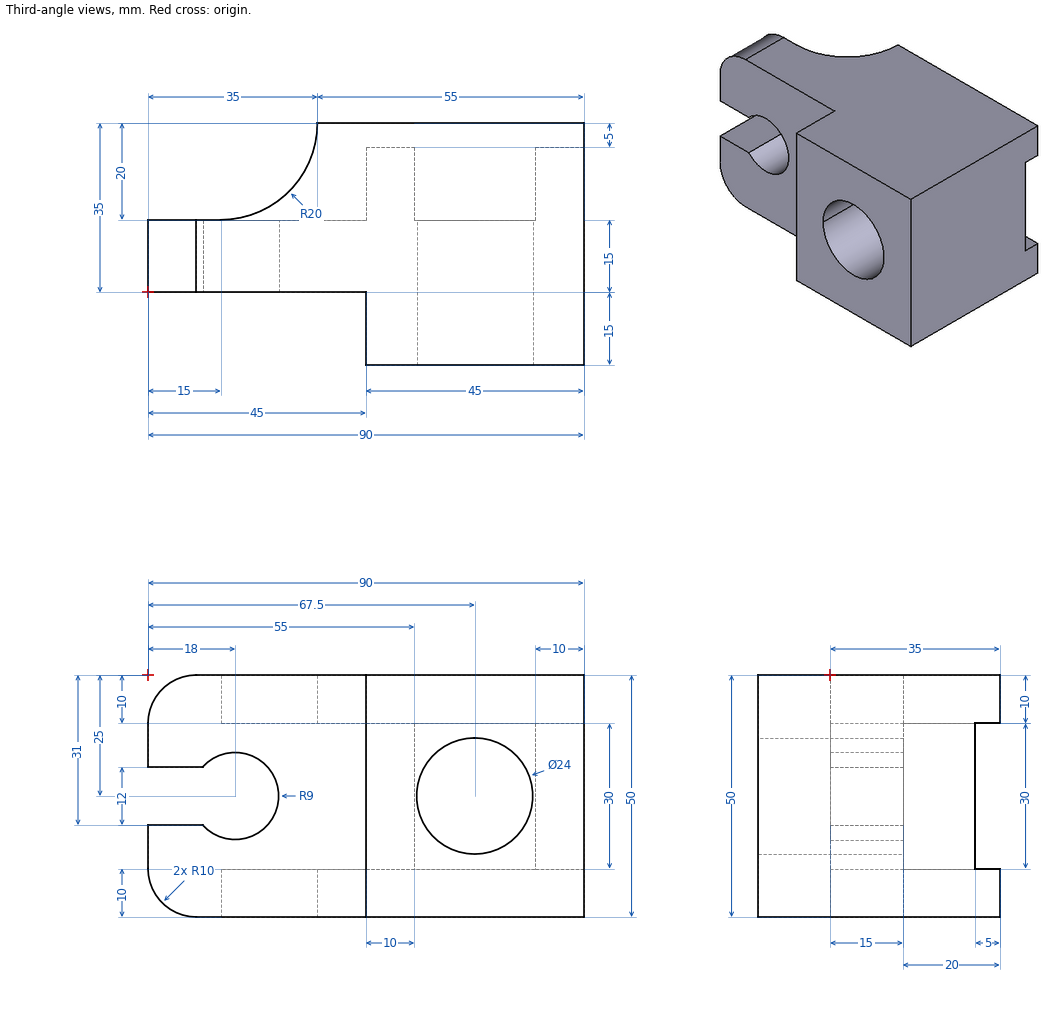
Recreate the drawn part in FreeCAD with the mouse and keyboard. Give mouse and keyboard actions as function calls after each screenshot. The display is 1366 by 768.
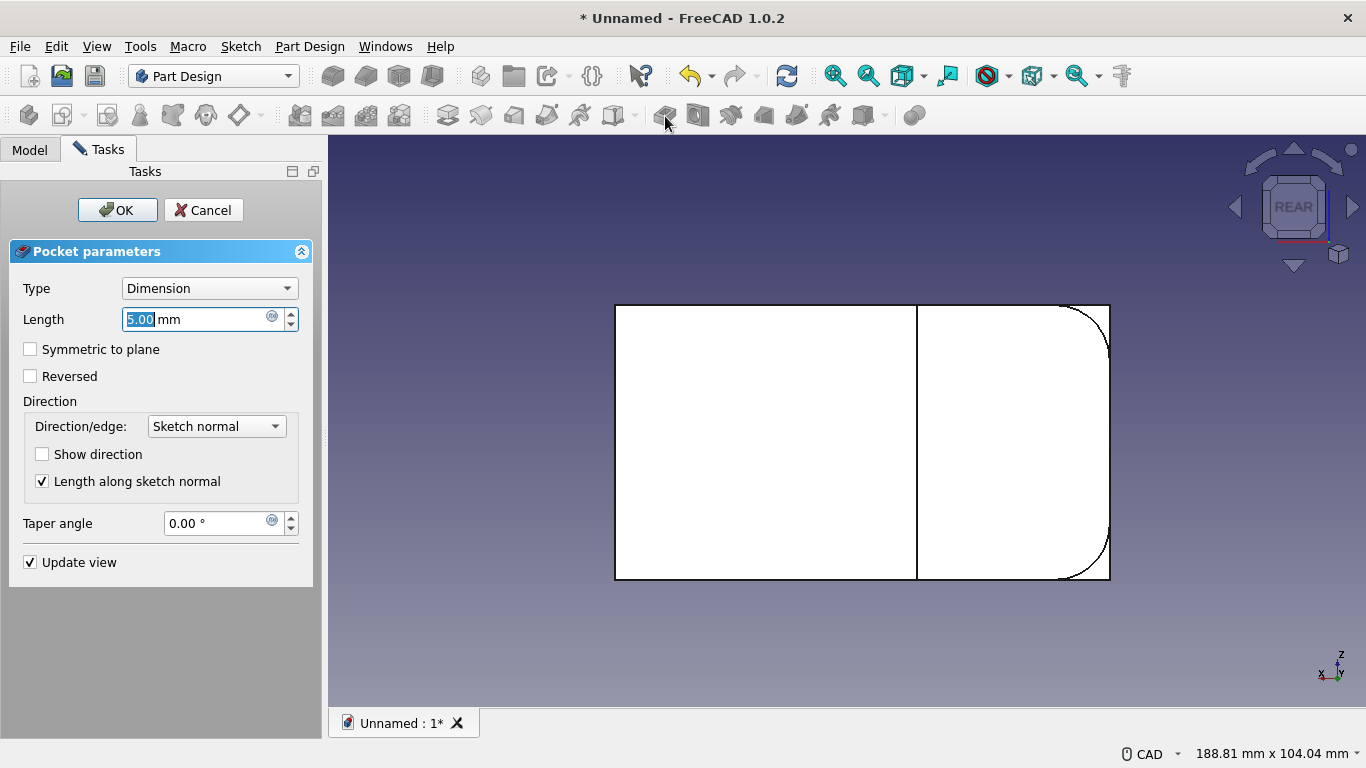
text(50)
key(Tab)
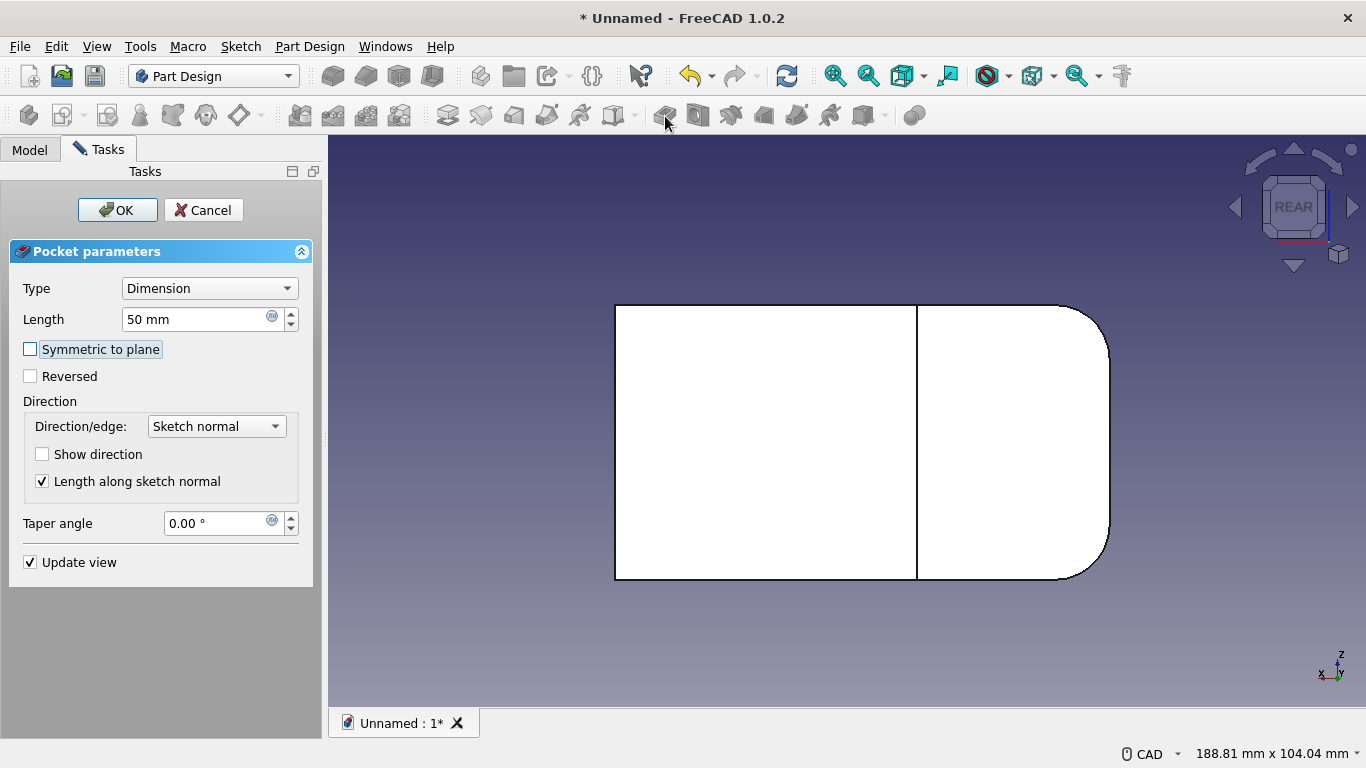
click(118, 210)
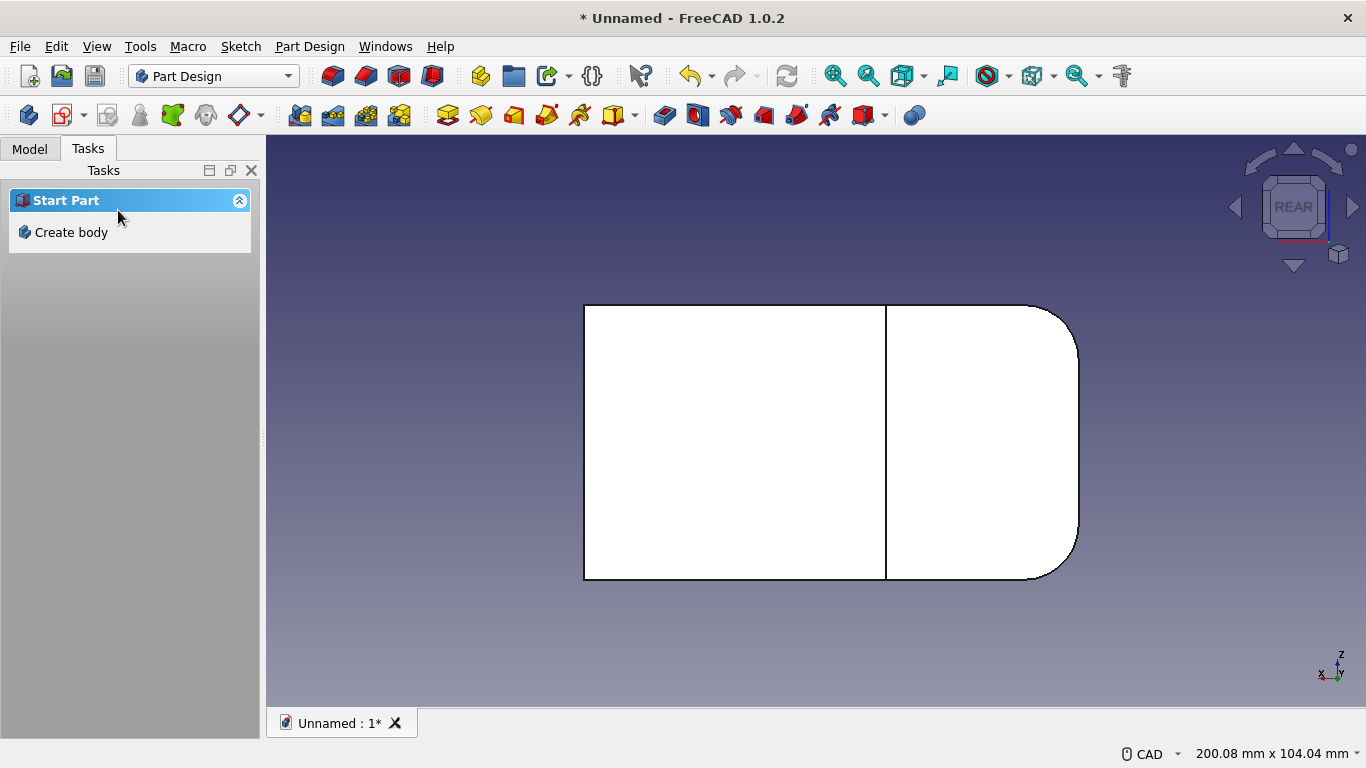
key(0)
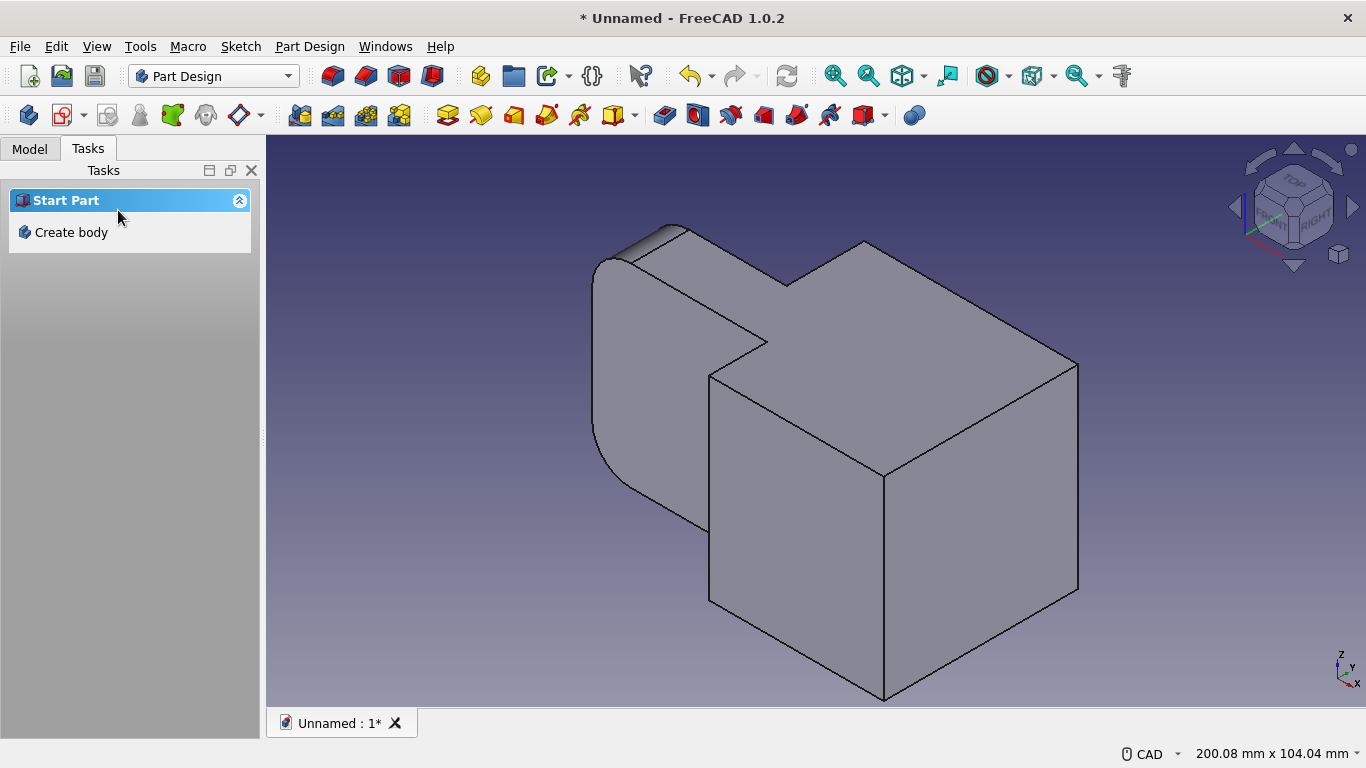
click(870, 355)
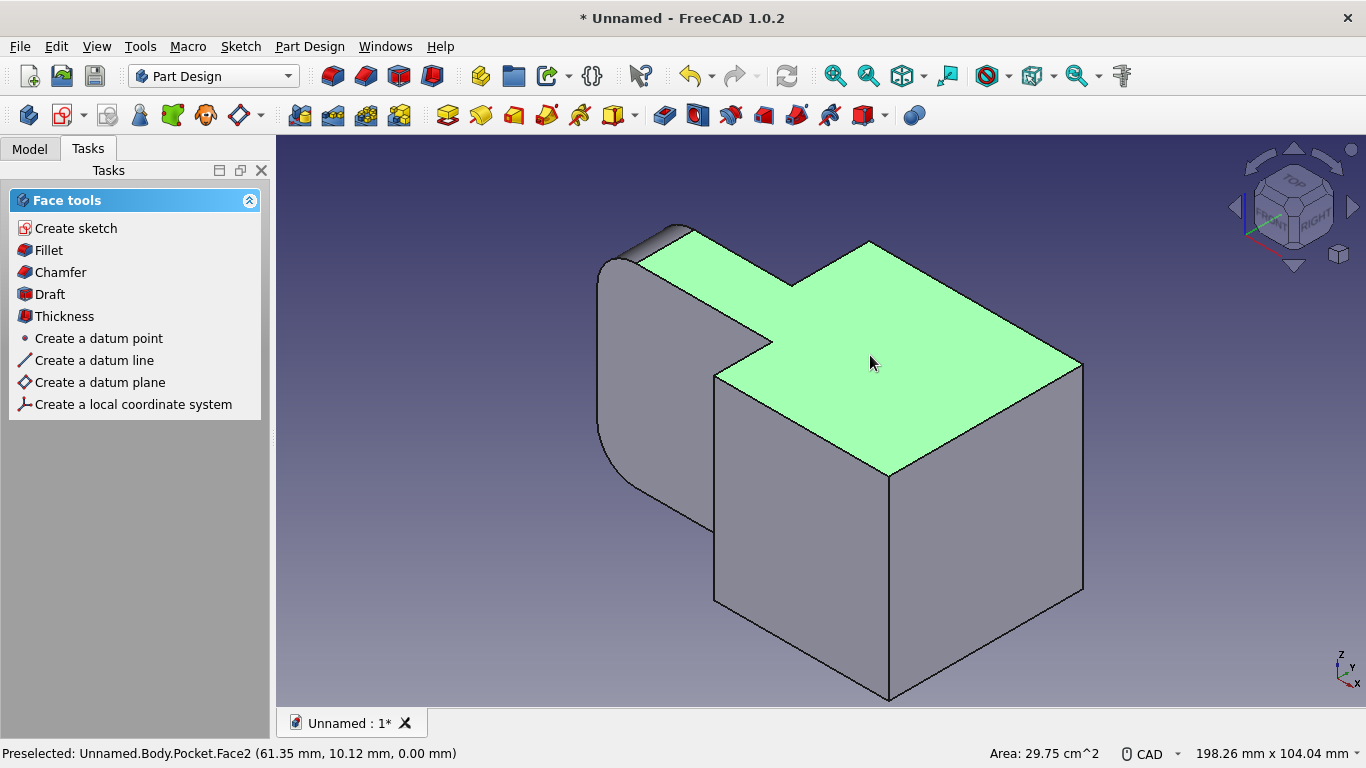
click(62, 116)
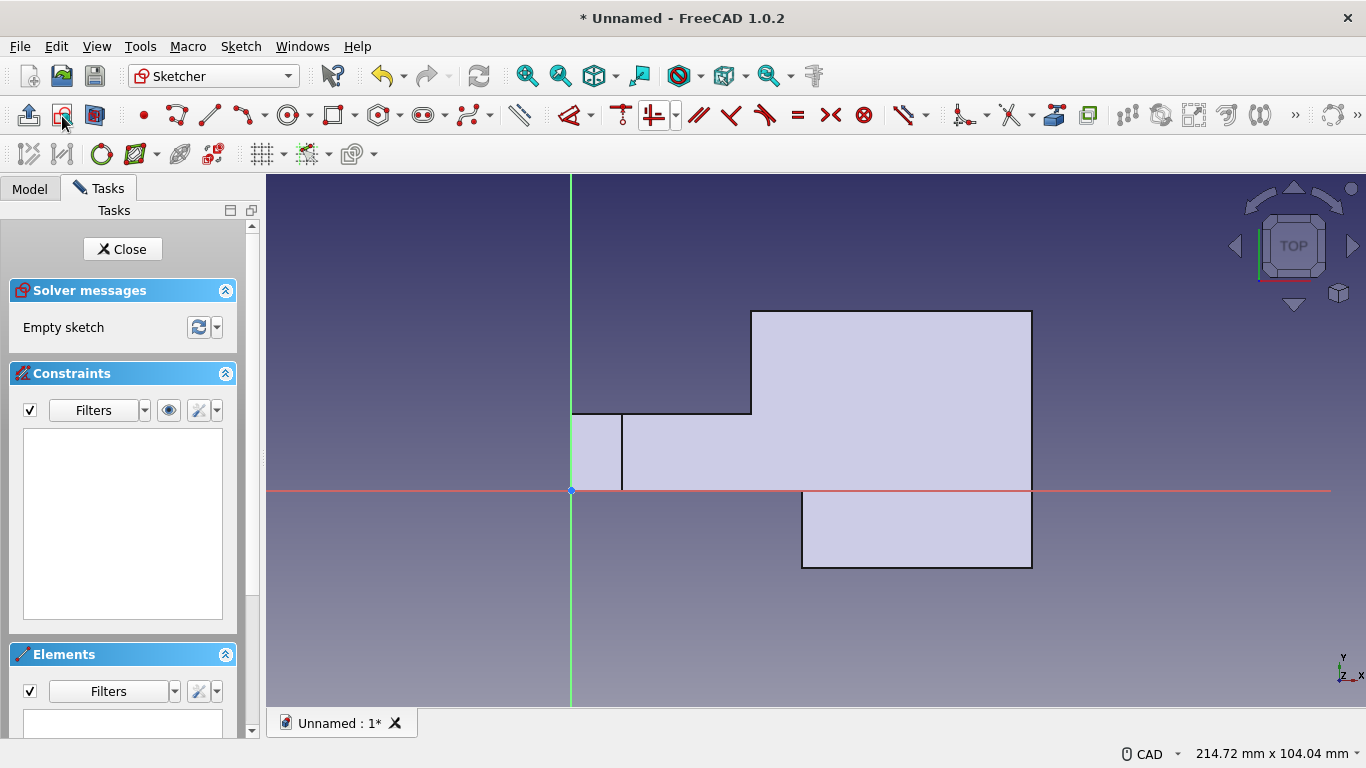
scroll(555, 353, up, 3)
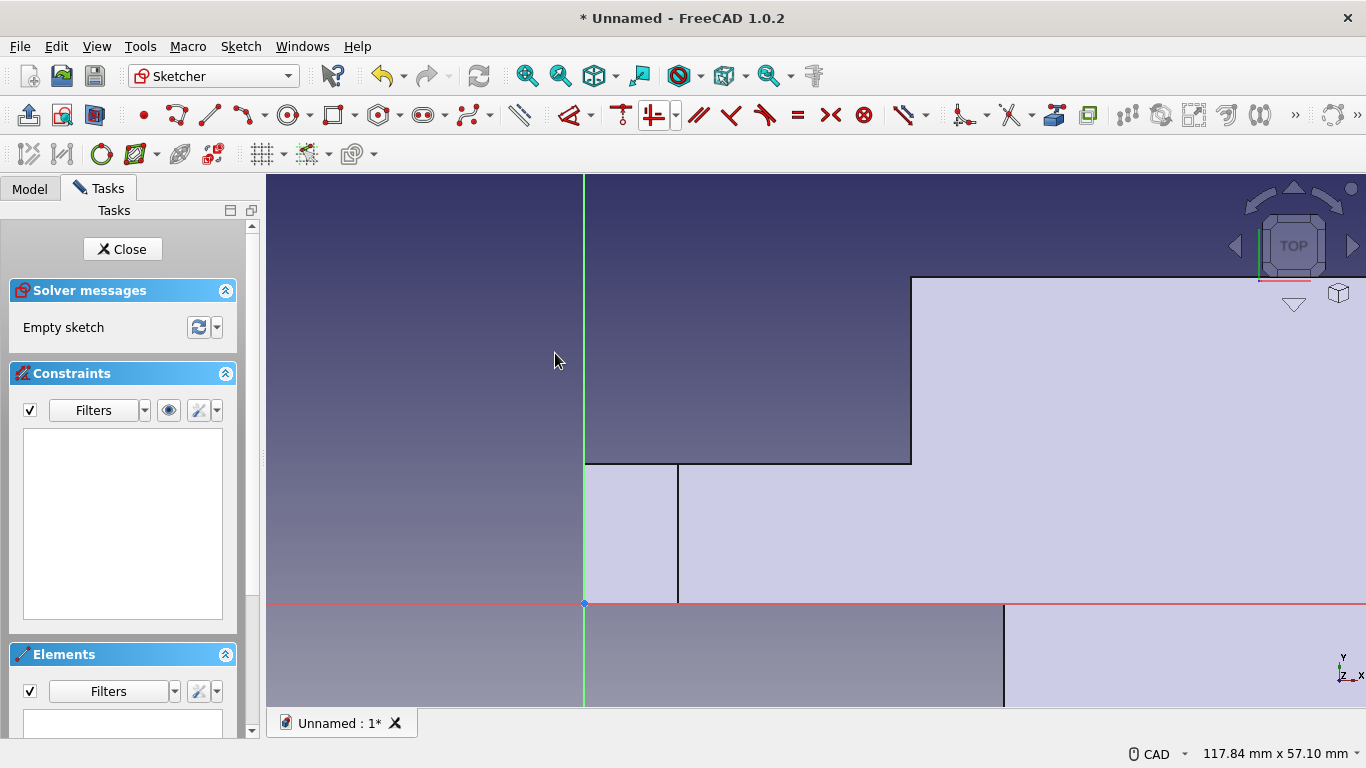
click(177, 116)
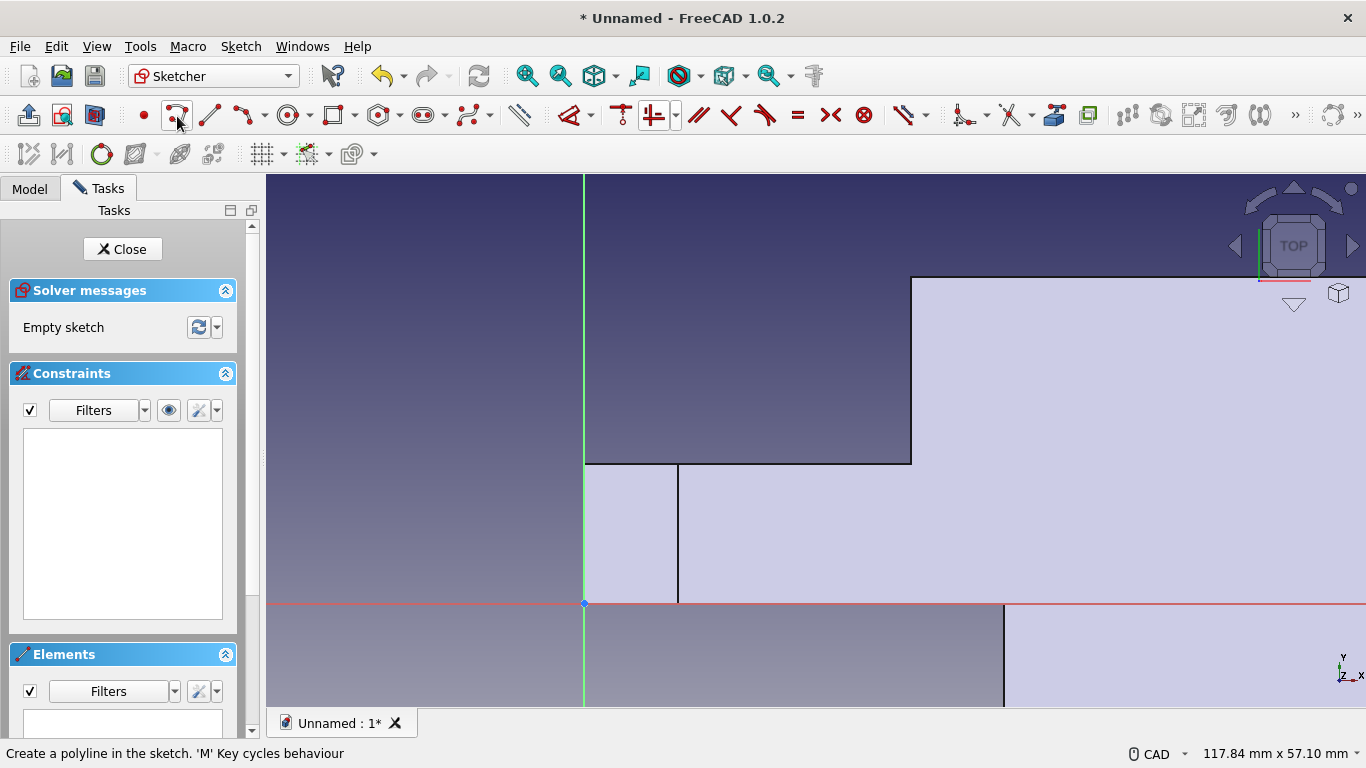
click(724, 464)
click(911, 464)
click(911, 277)
right_click(911, 277)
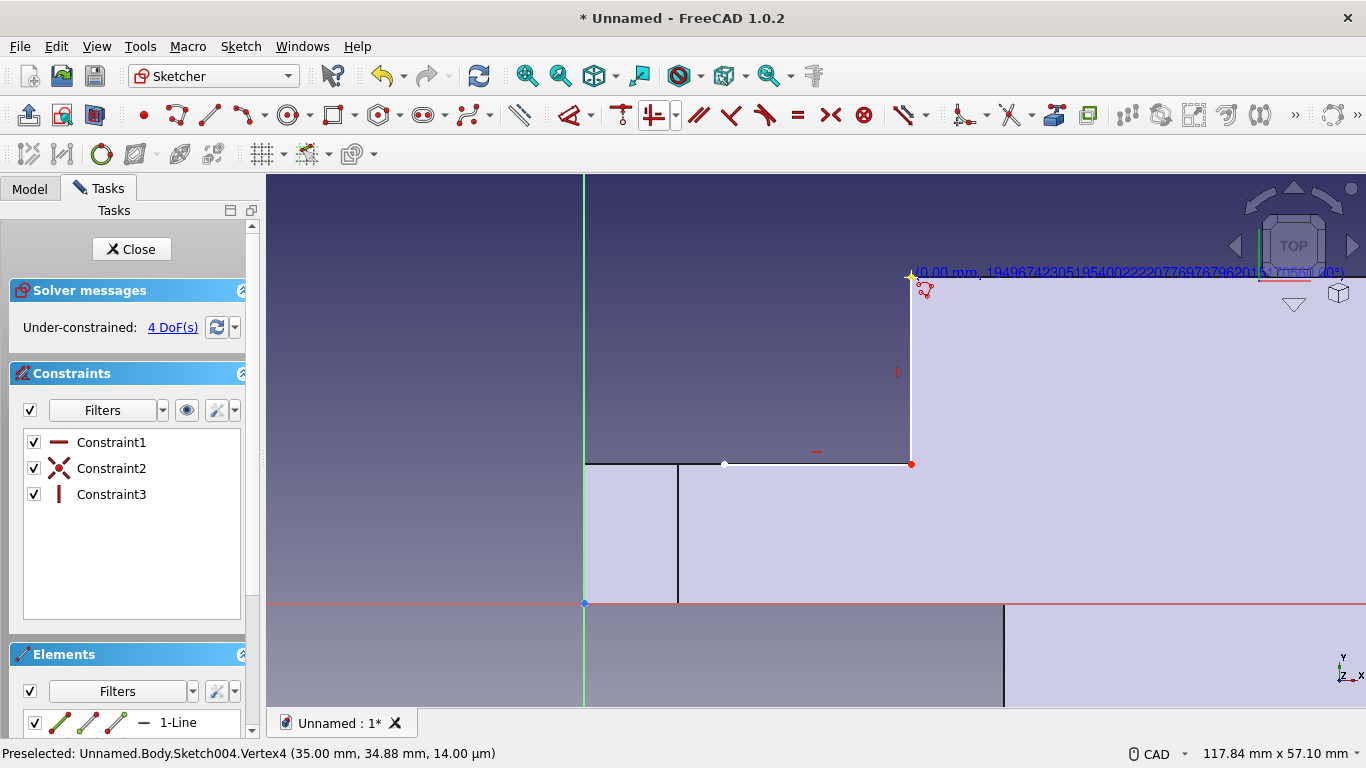
click(242, 116)